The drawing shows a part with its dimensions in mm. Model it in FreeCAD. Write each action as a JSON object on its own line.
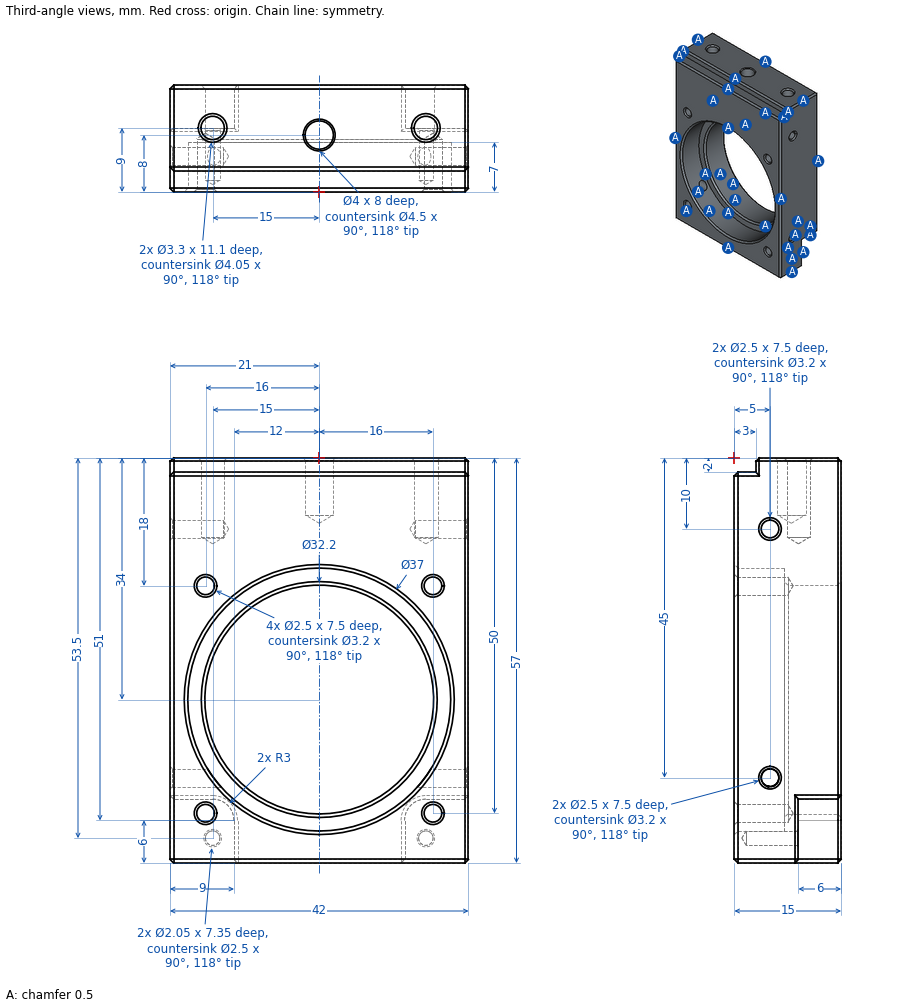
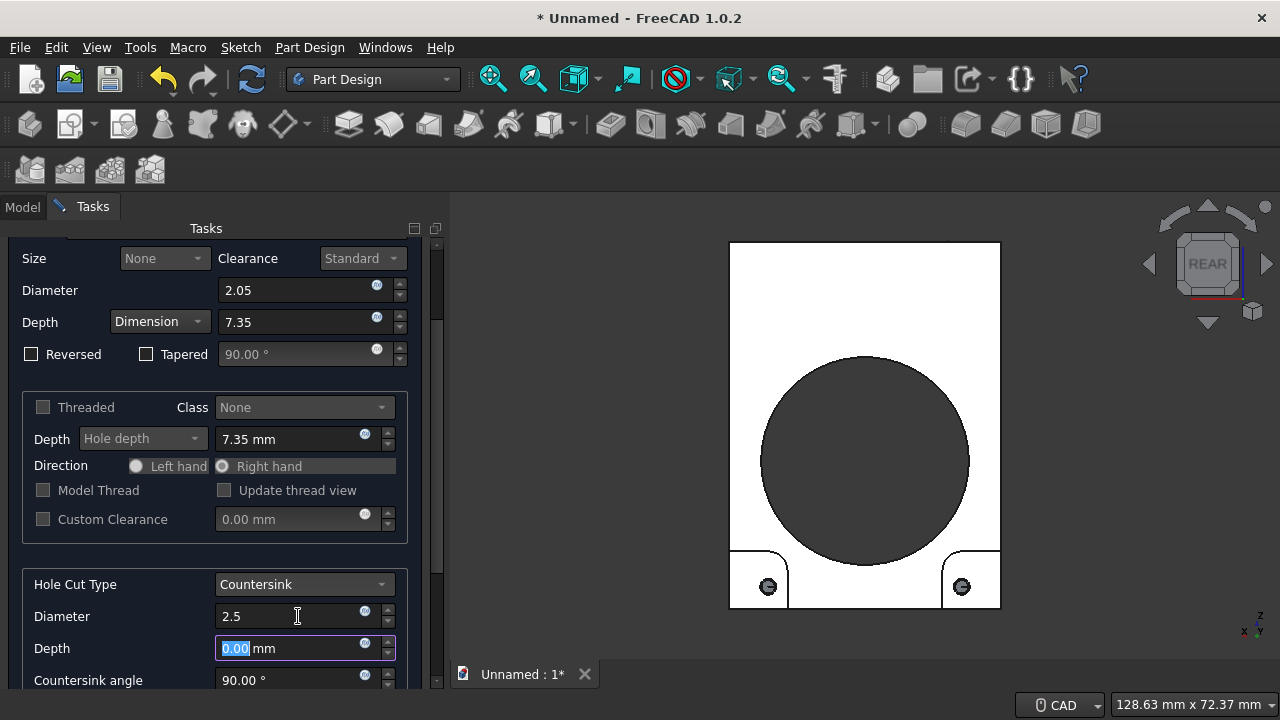
{"action": "scroll", "coordinate": [437, 463], "scroll_direction": "up", "scroll_amount": 3}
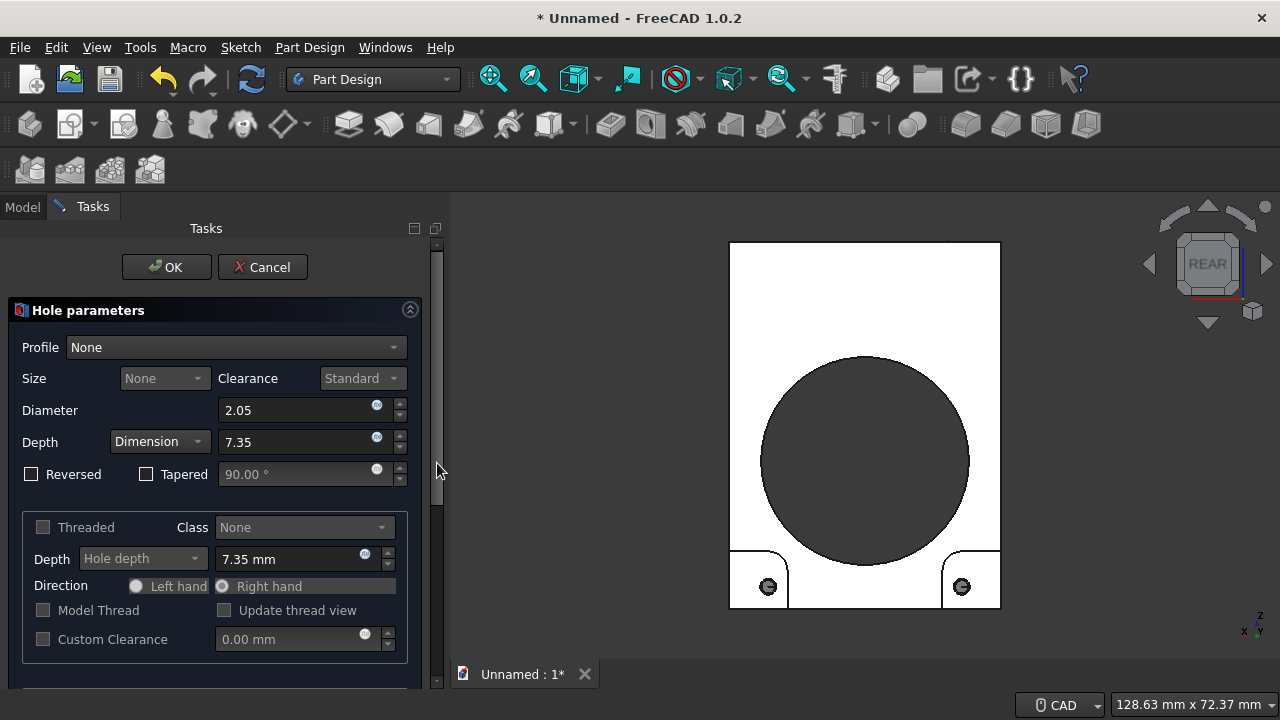
{"action": "left_click", "coordinate": [167, 267]}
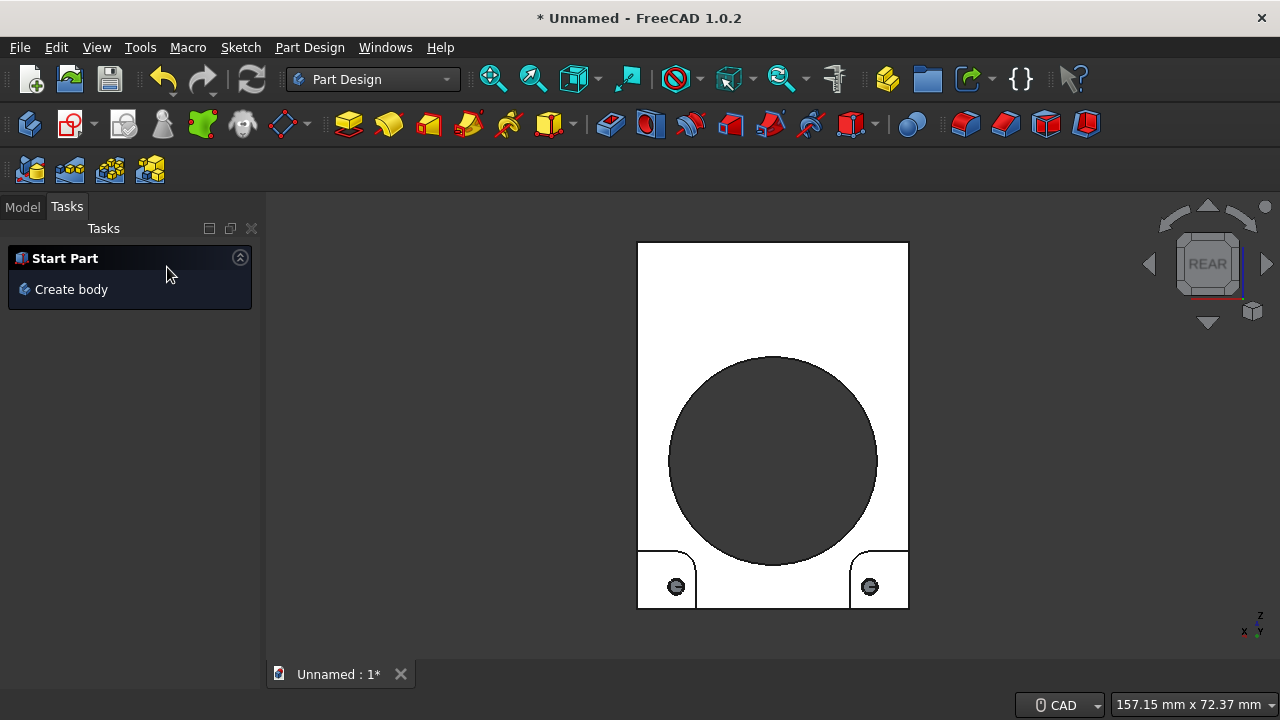
{"action": "key", "text": "6"}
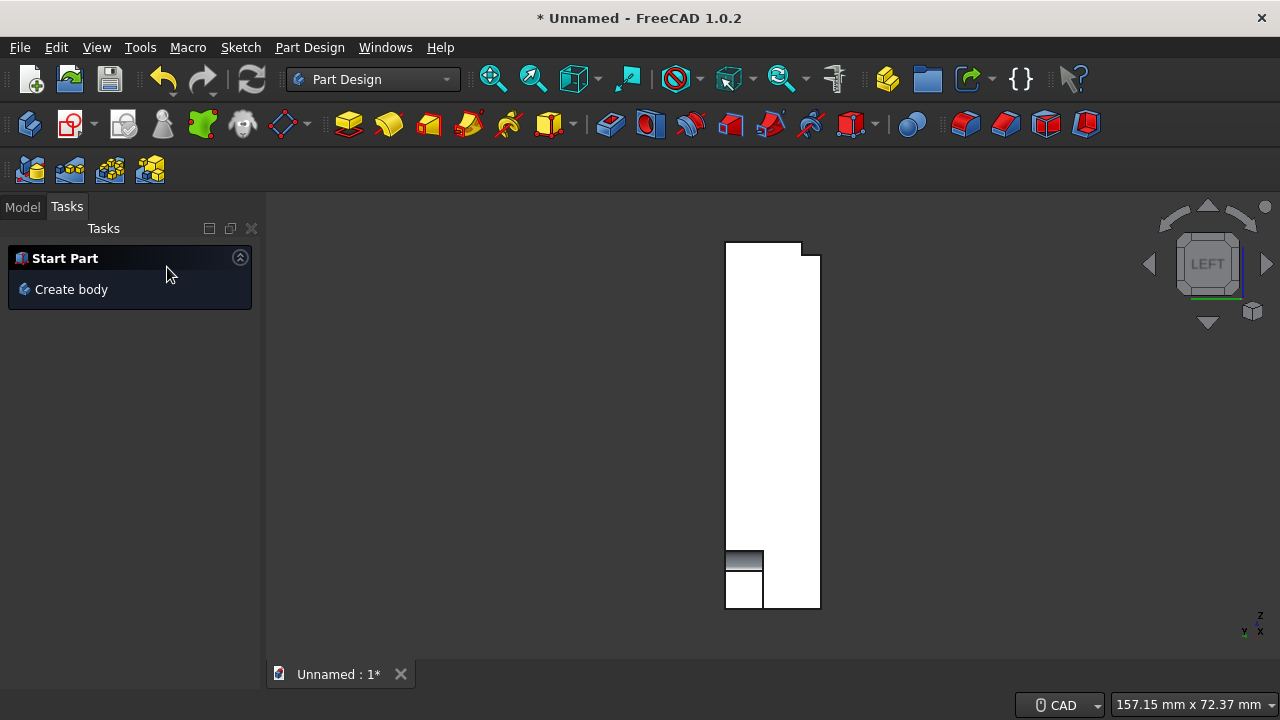
{"action": "left_click", "coordinate": [773, 319]}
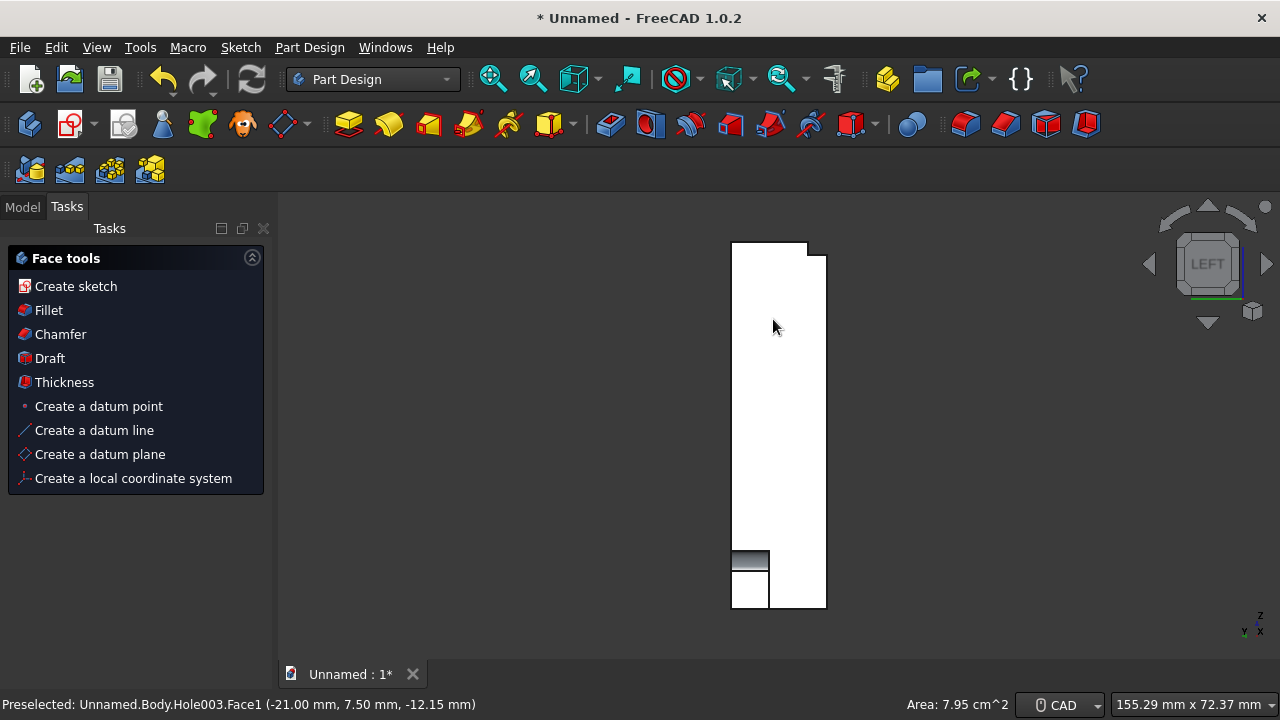
{"action": "left_click", "coordinate": [70, 124]}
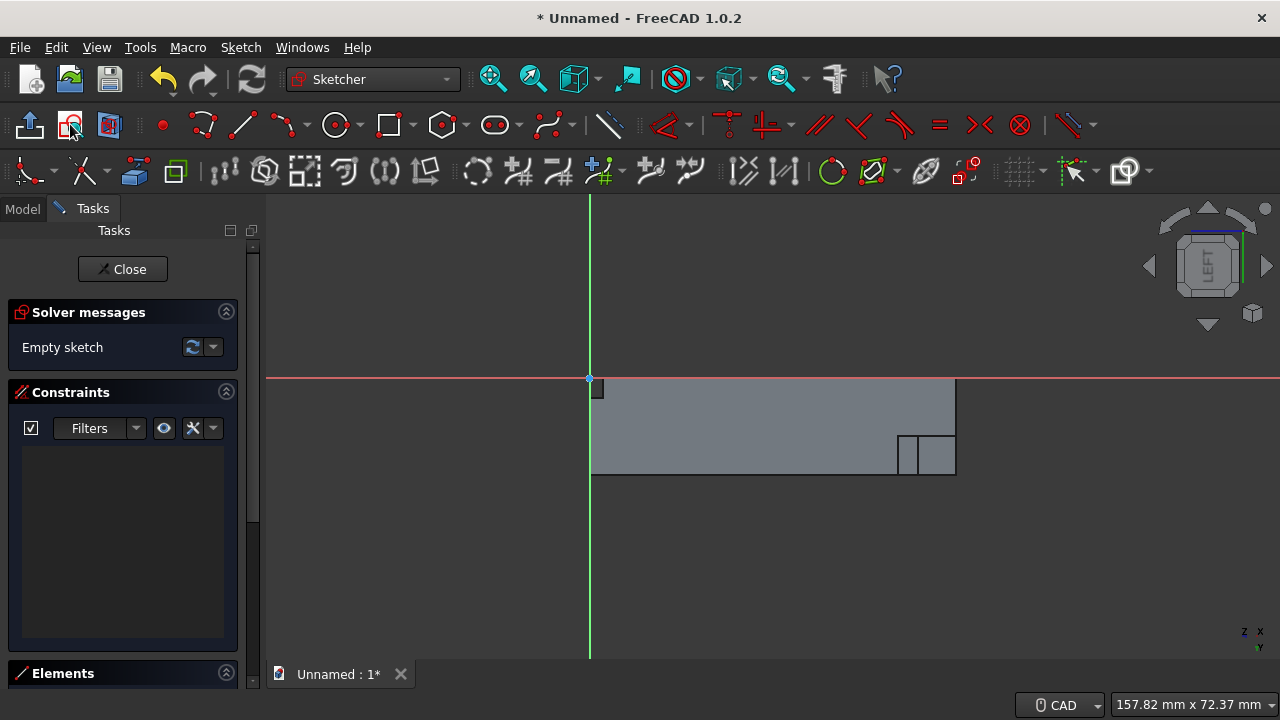
{"action": "scroll", "coordinate": [780, 364], "scroll_direction": "up", "scroll_amount": 3}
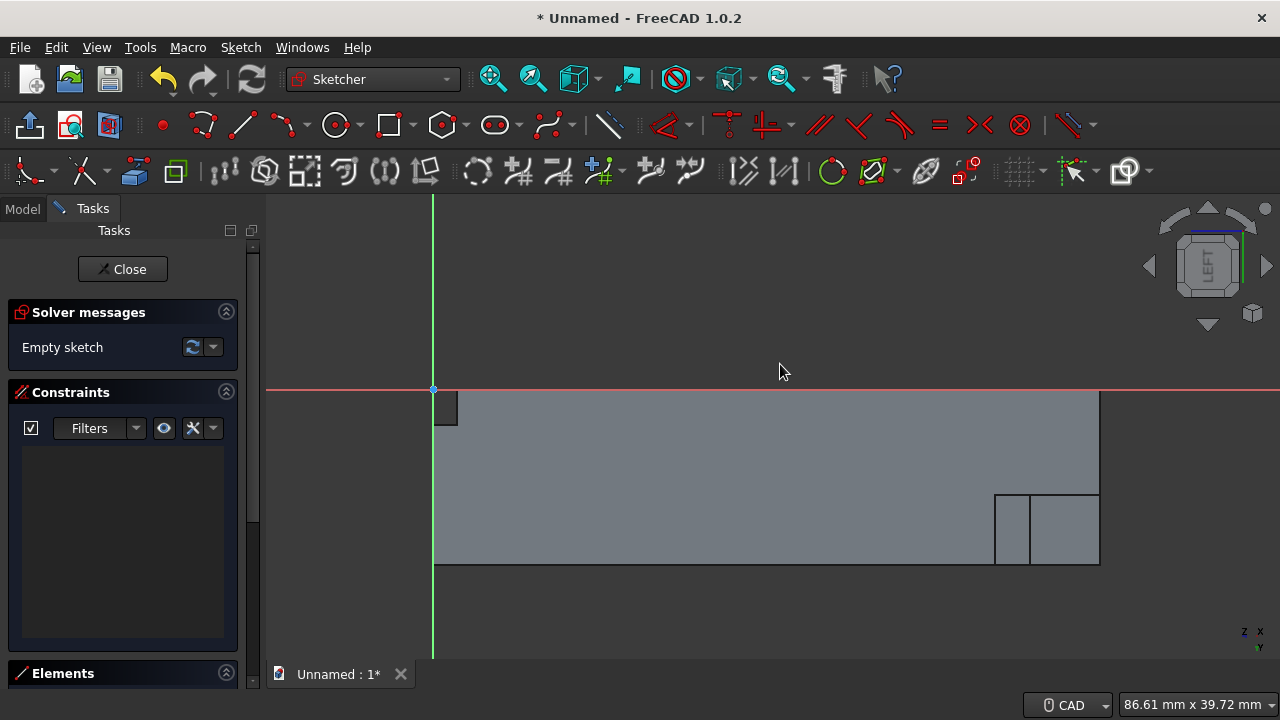
{"action": "left_click", "coordinate": [336, 126]}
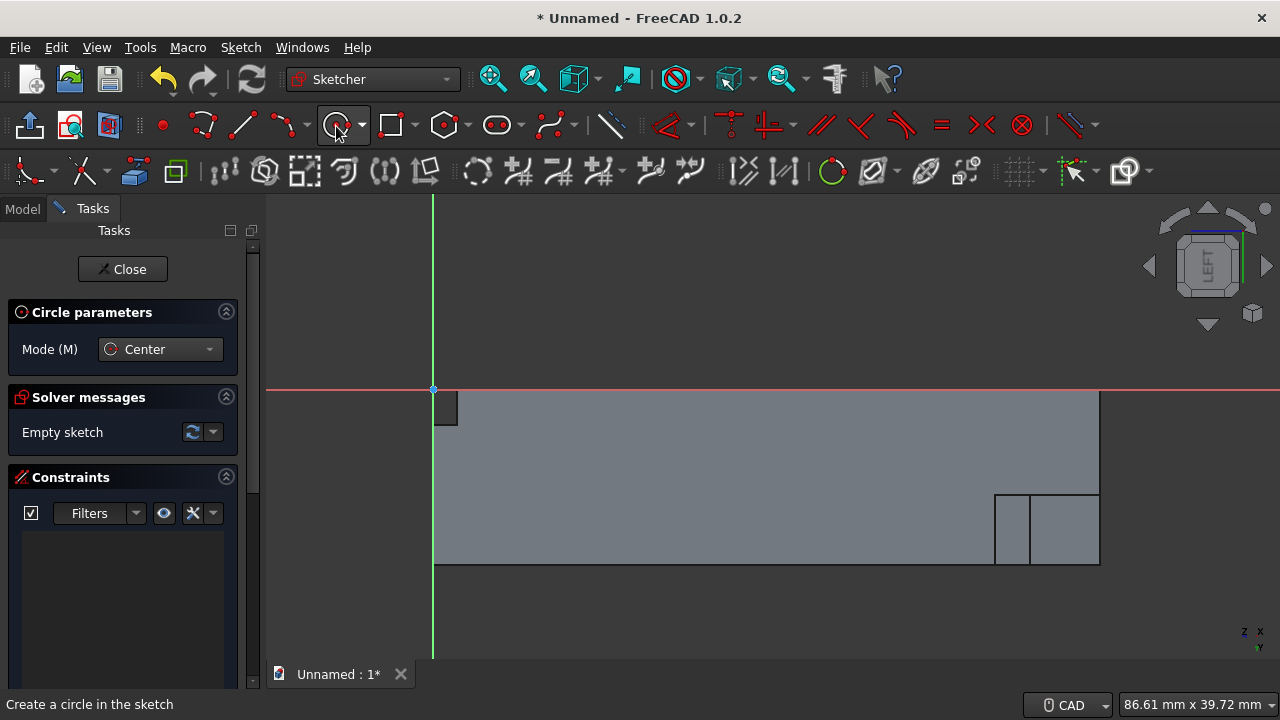
{"action": "scroll", "coordinate": [960, 448], "scroll_direction": "up", "scroll_amount": 3}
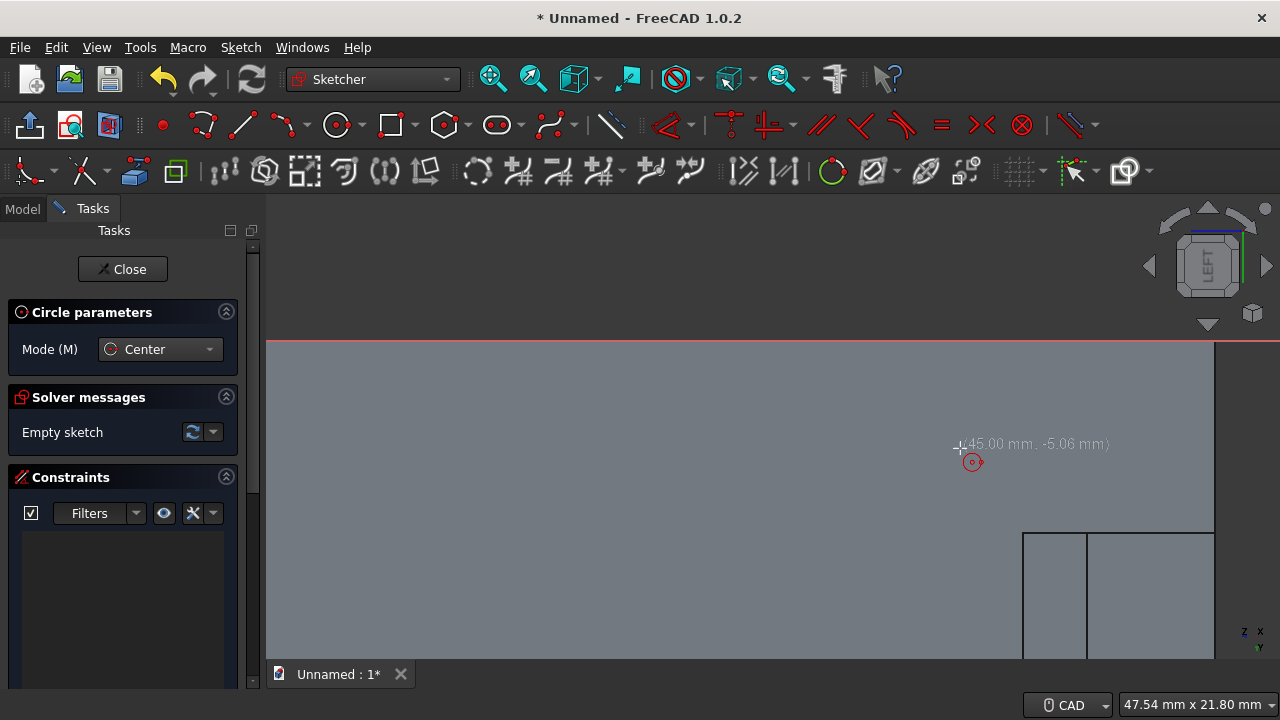
{"action": "left_click", "coordinate": [959, 448]}
{"action": "mouse_move", "coordinate": [978, 429]}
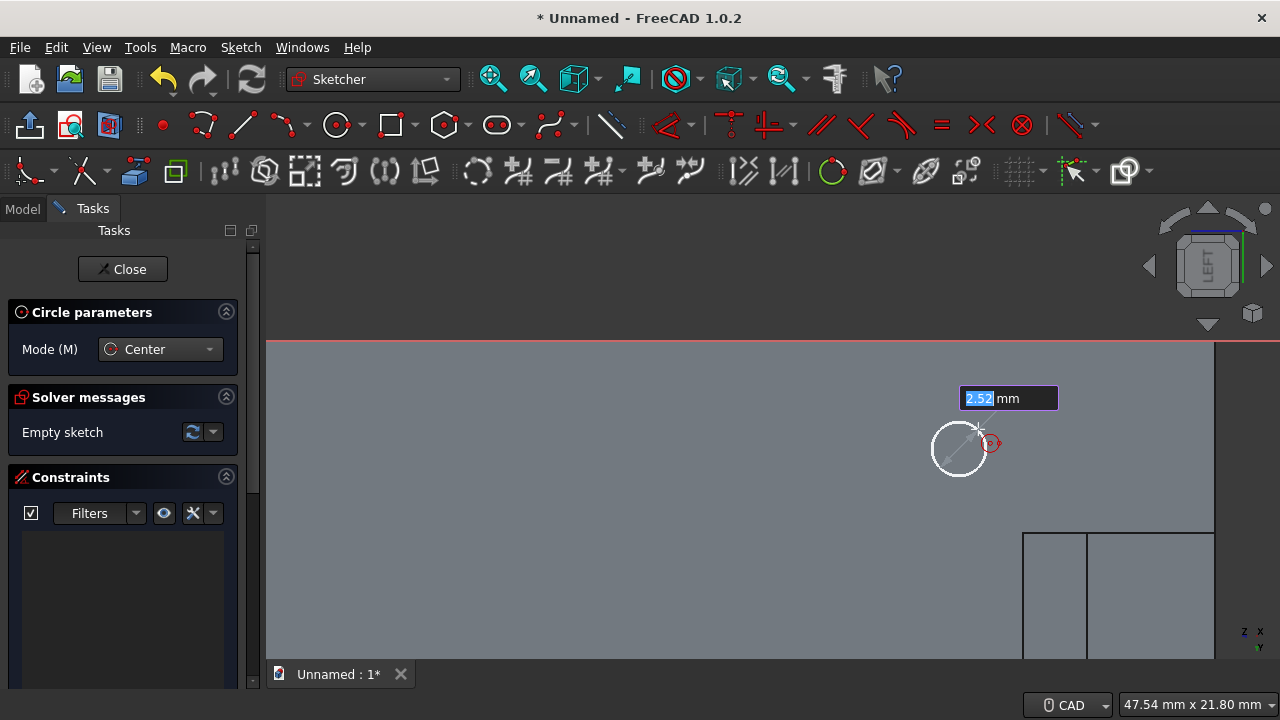
{"action": "type", "text": "2.5"}
{"action": "key", "text": "Return"}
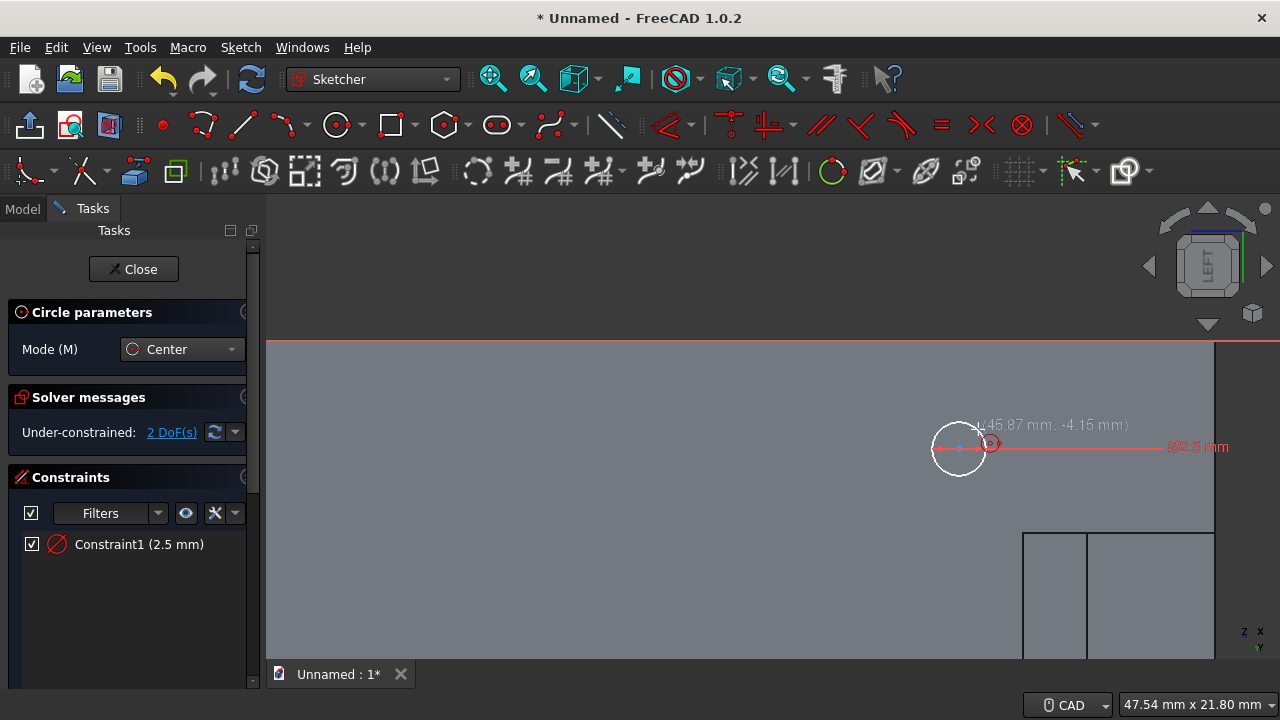
{"action": "scroll", "coordinate": [962, 449], "scroll_direction": "down", "scroll_amount": 3}